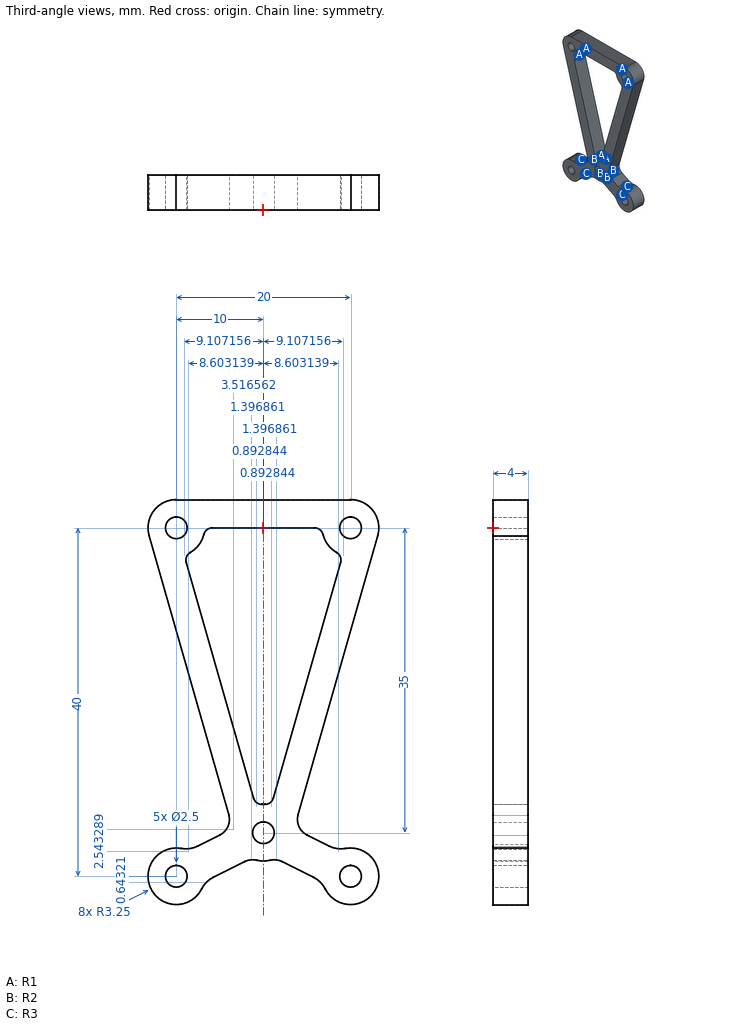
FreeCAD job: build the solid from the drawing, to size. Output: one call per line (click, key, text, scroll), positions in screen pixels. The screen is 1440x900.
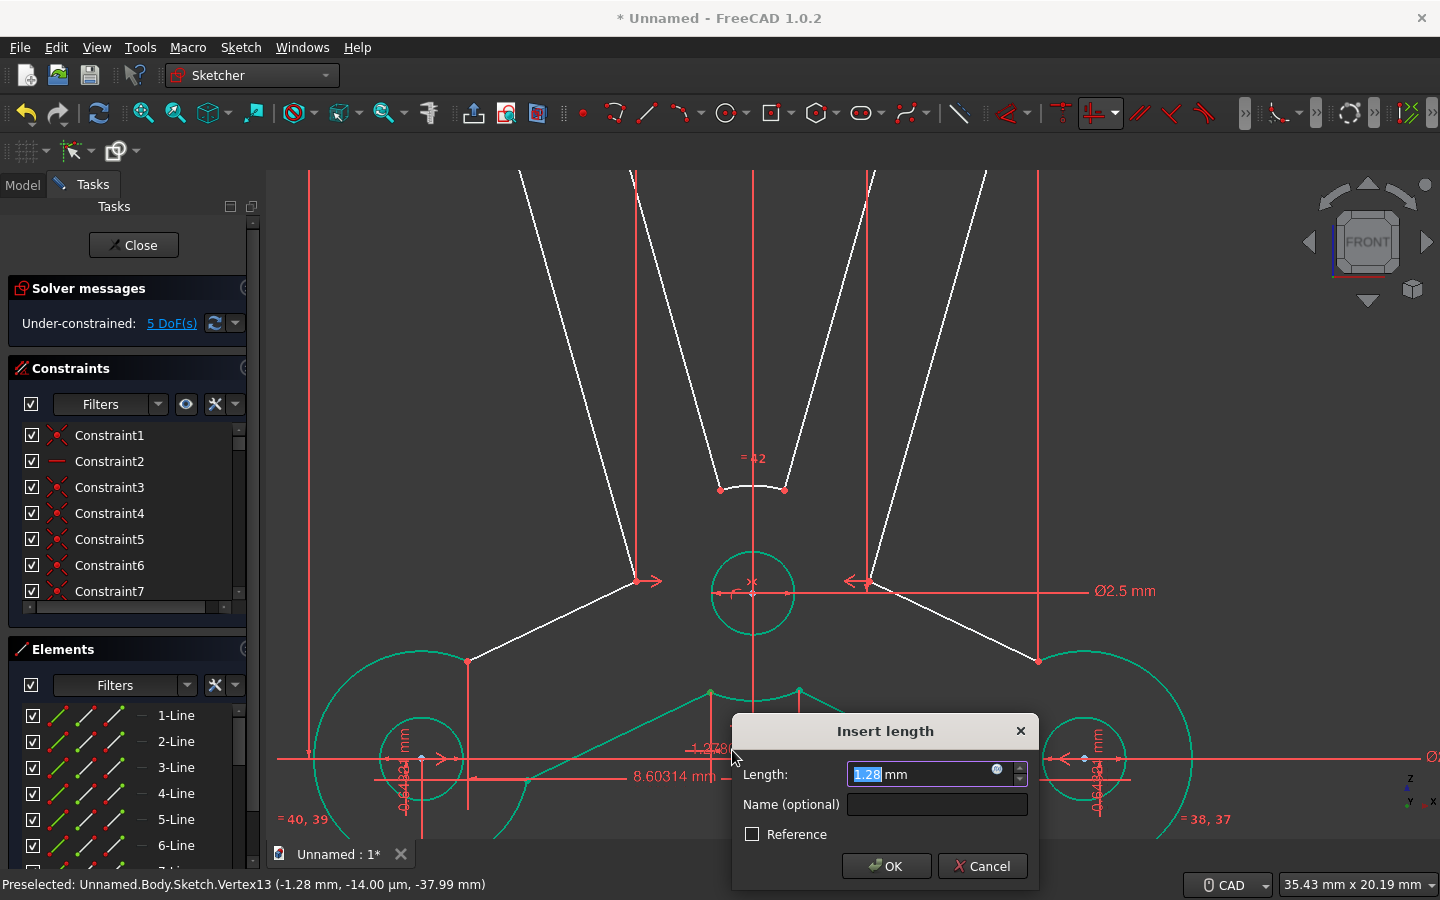
text(1.396861)
key(Return)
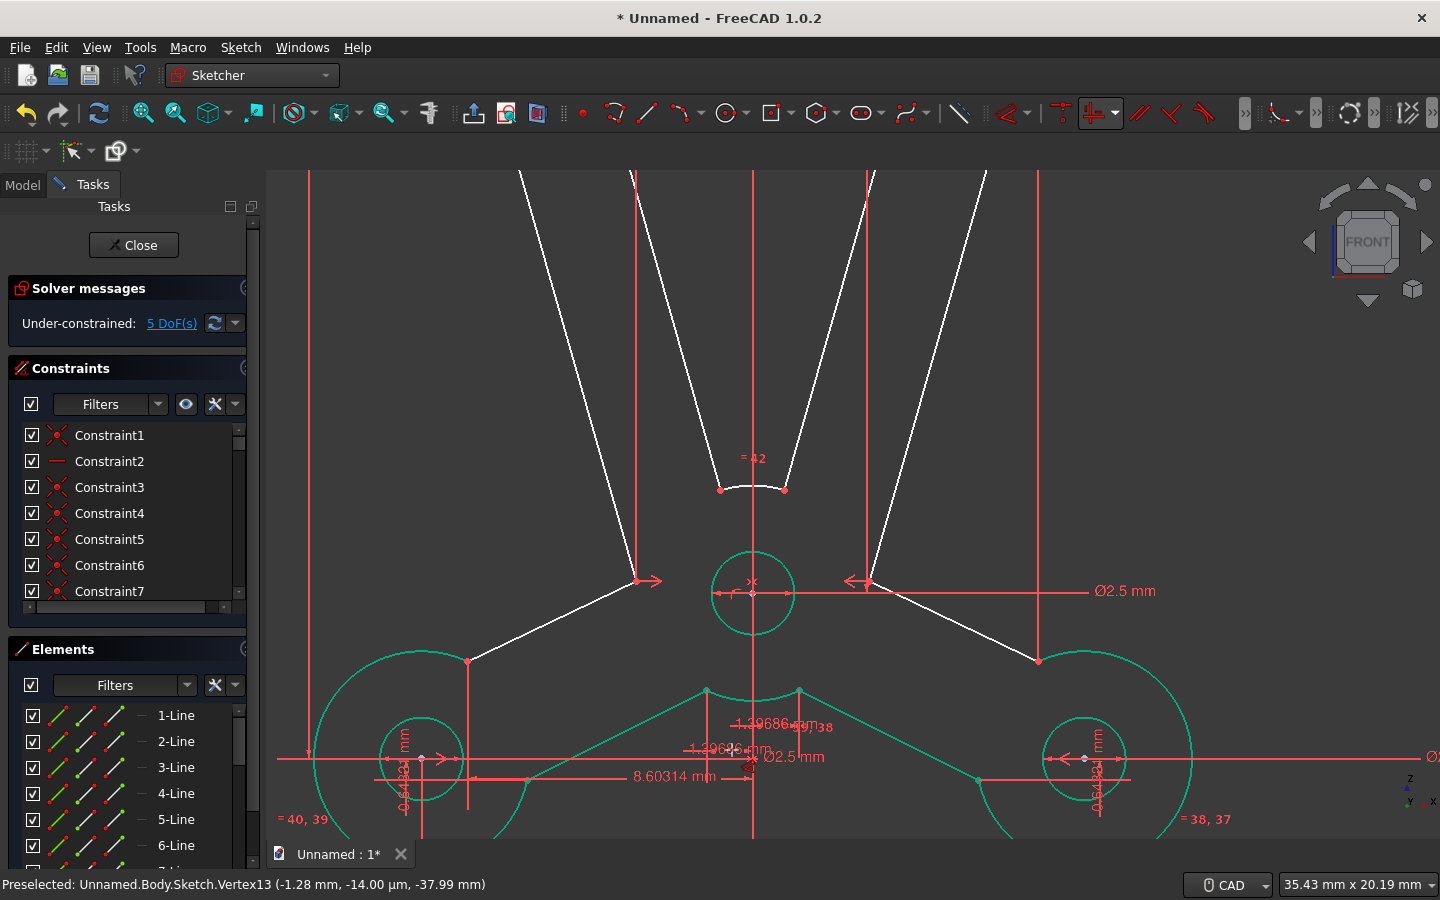
scroll(784, 490, up, 2)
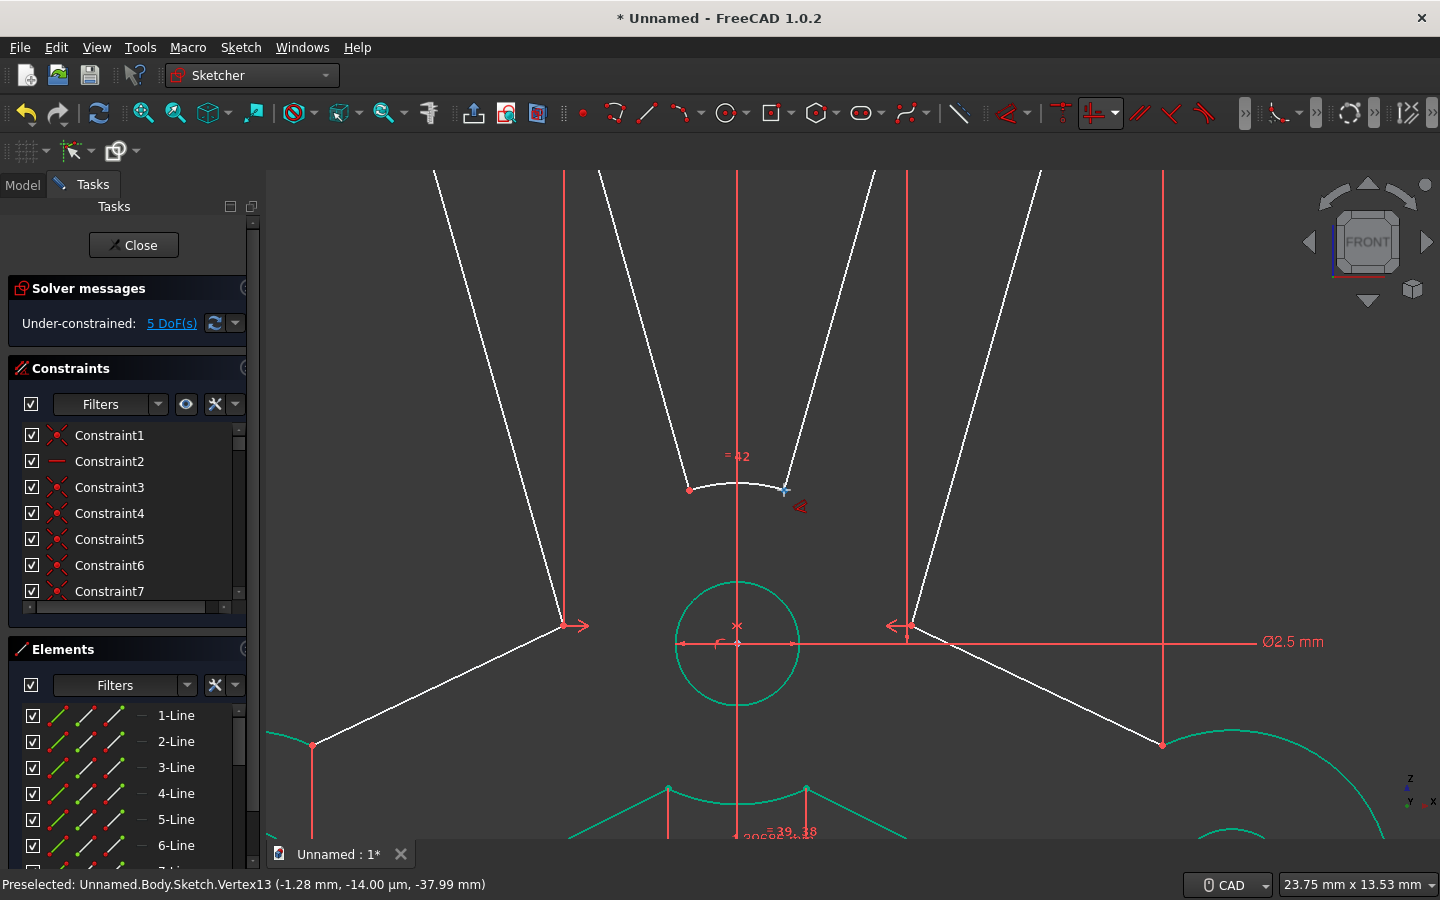
click(784, 490)
click(761, 524)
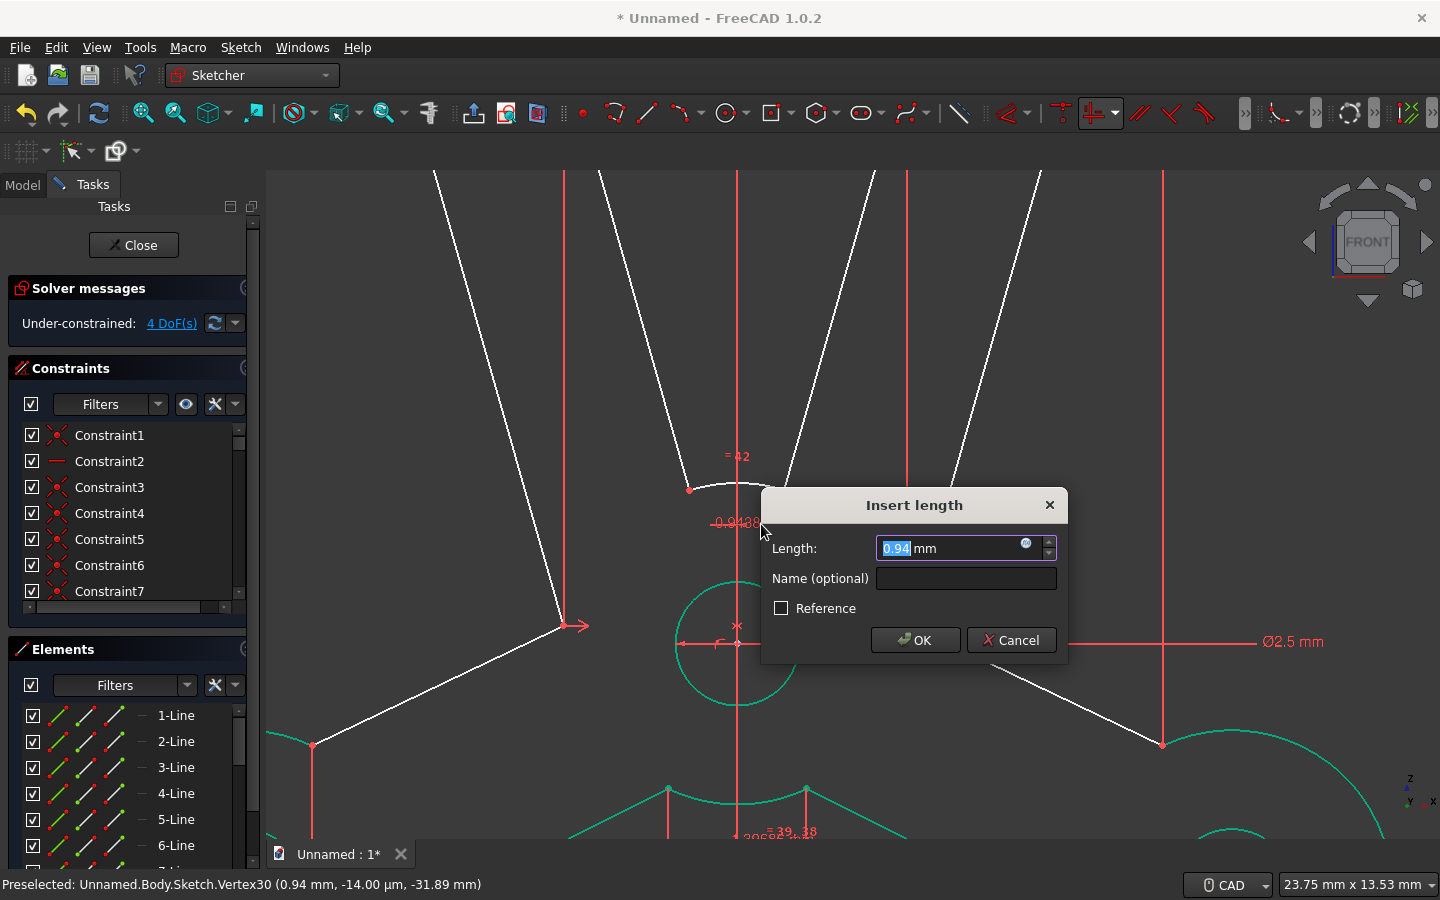
text(0.892844)
key(Return)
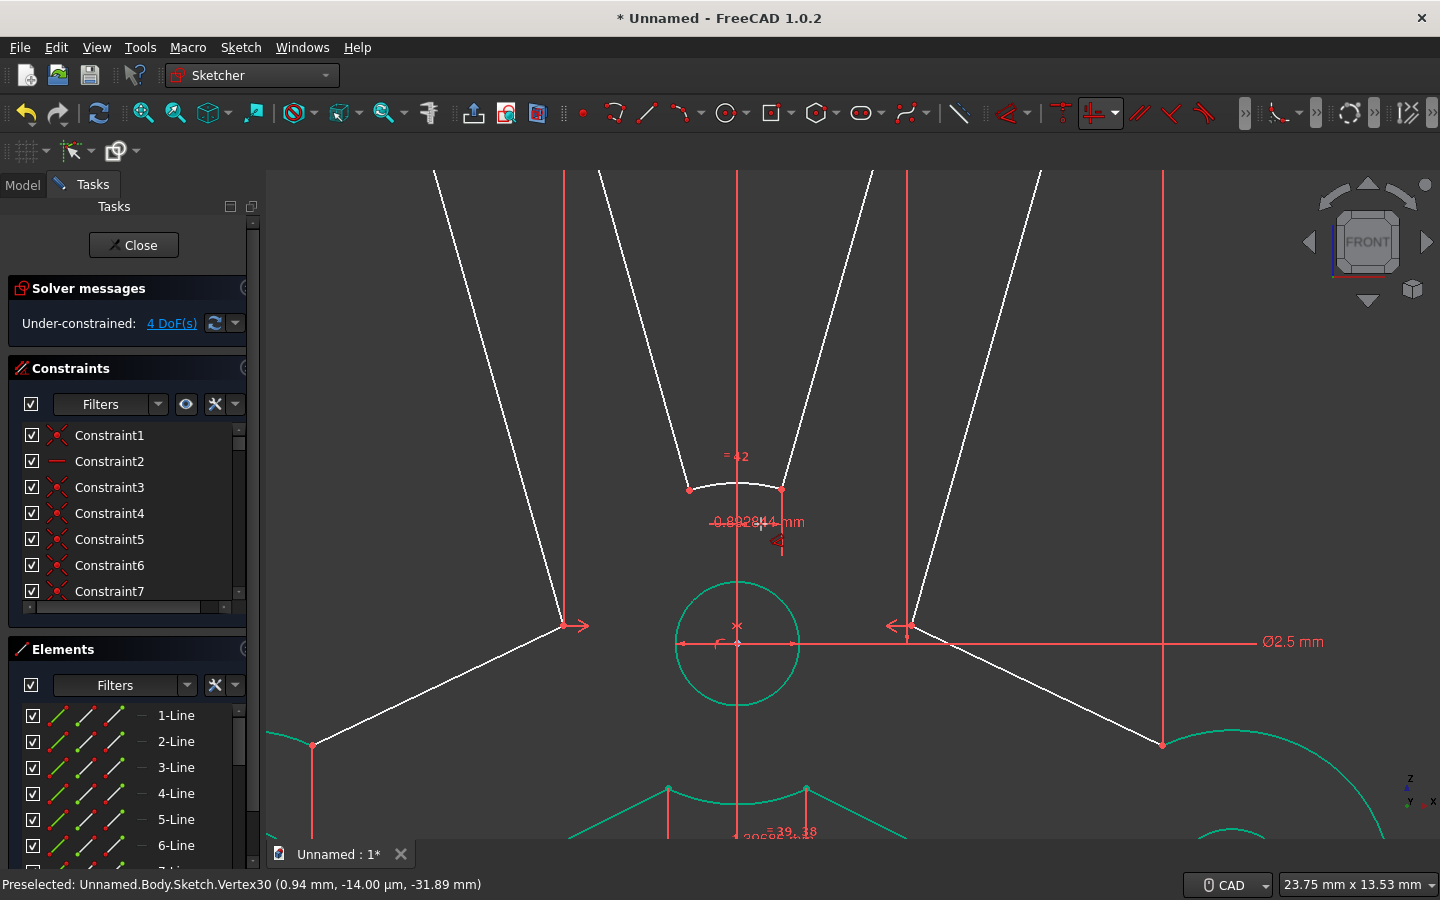
scroll(796, 668, down, 8)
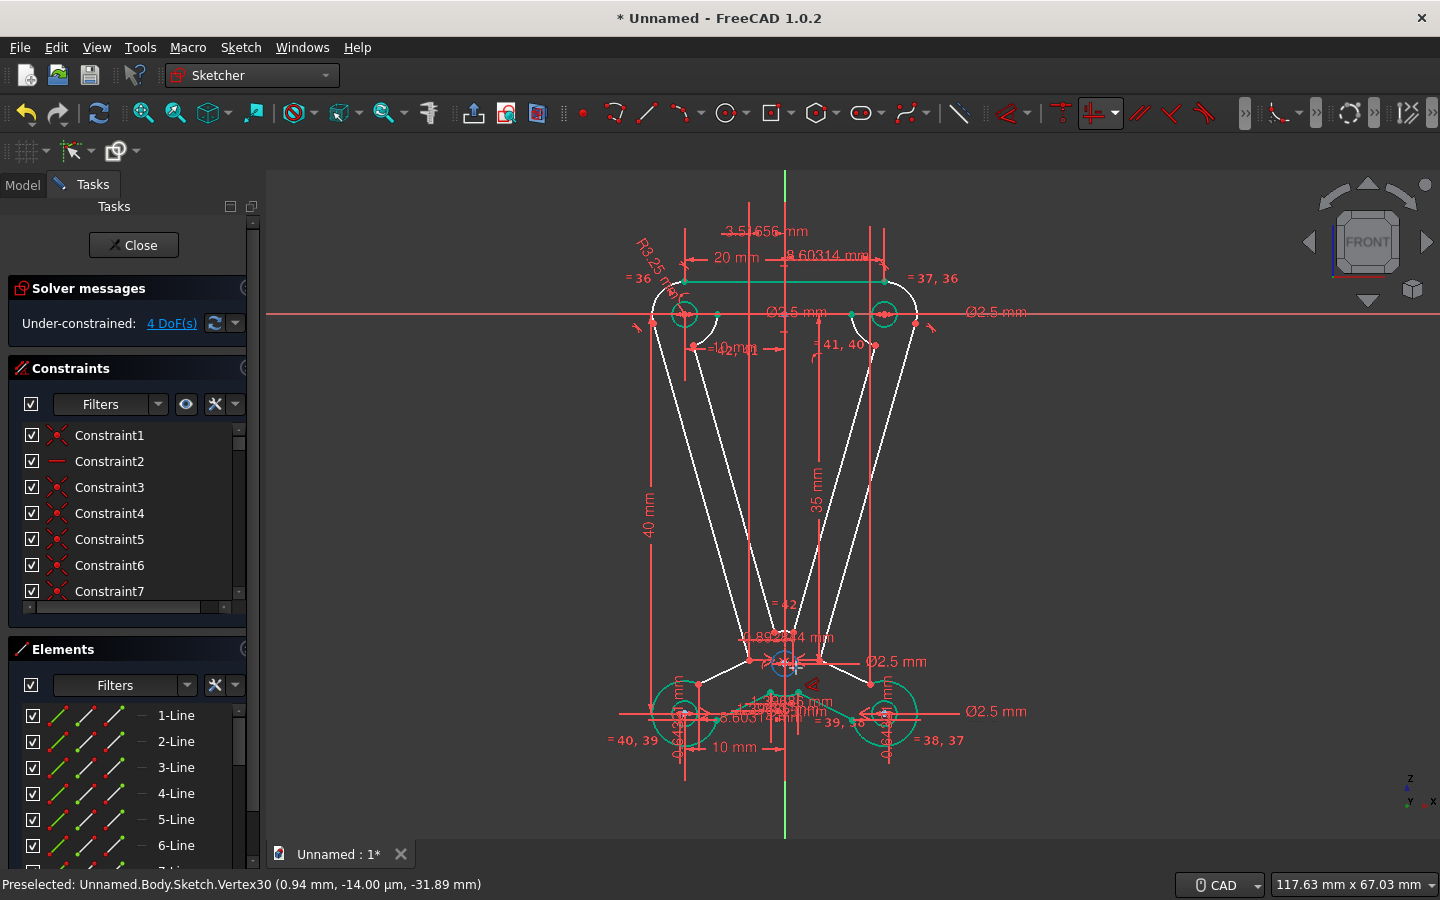
click(876, 346)
click(830, 380)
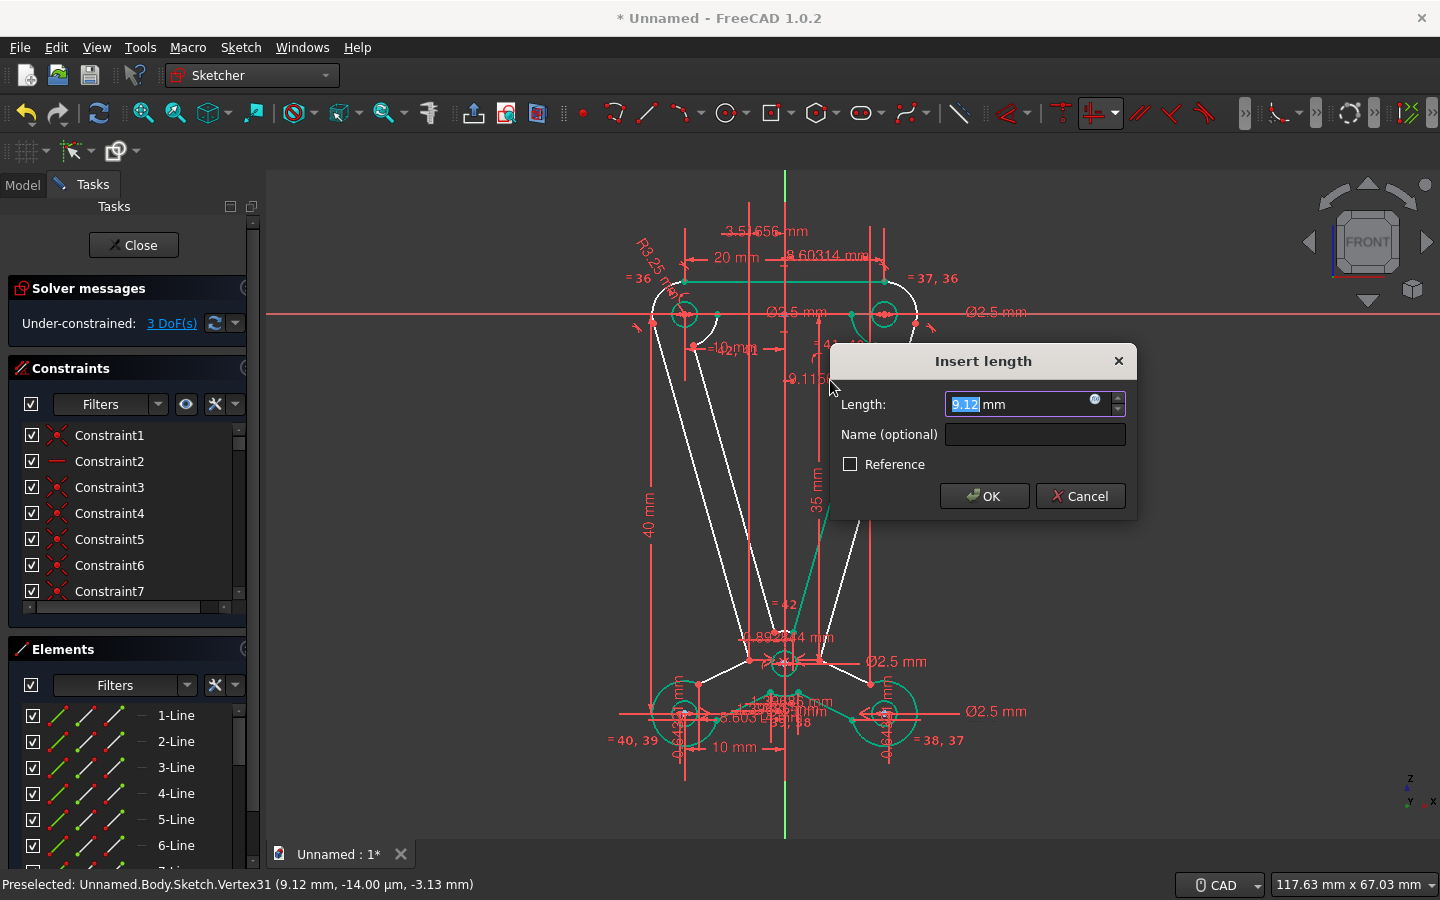
text(9.107156)
key(Return)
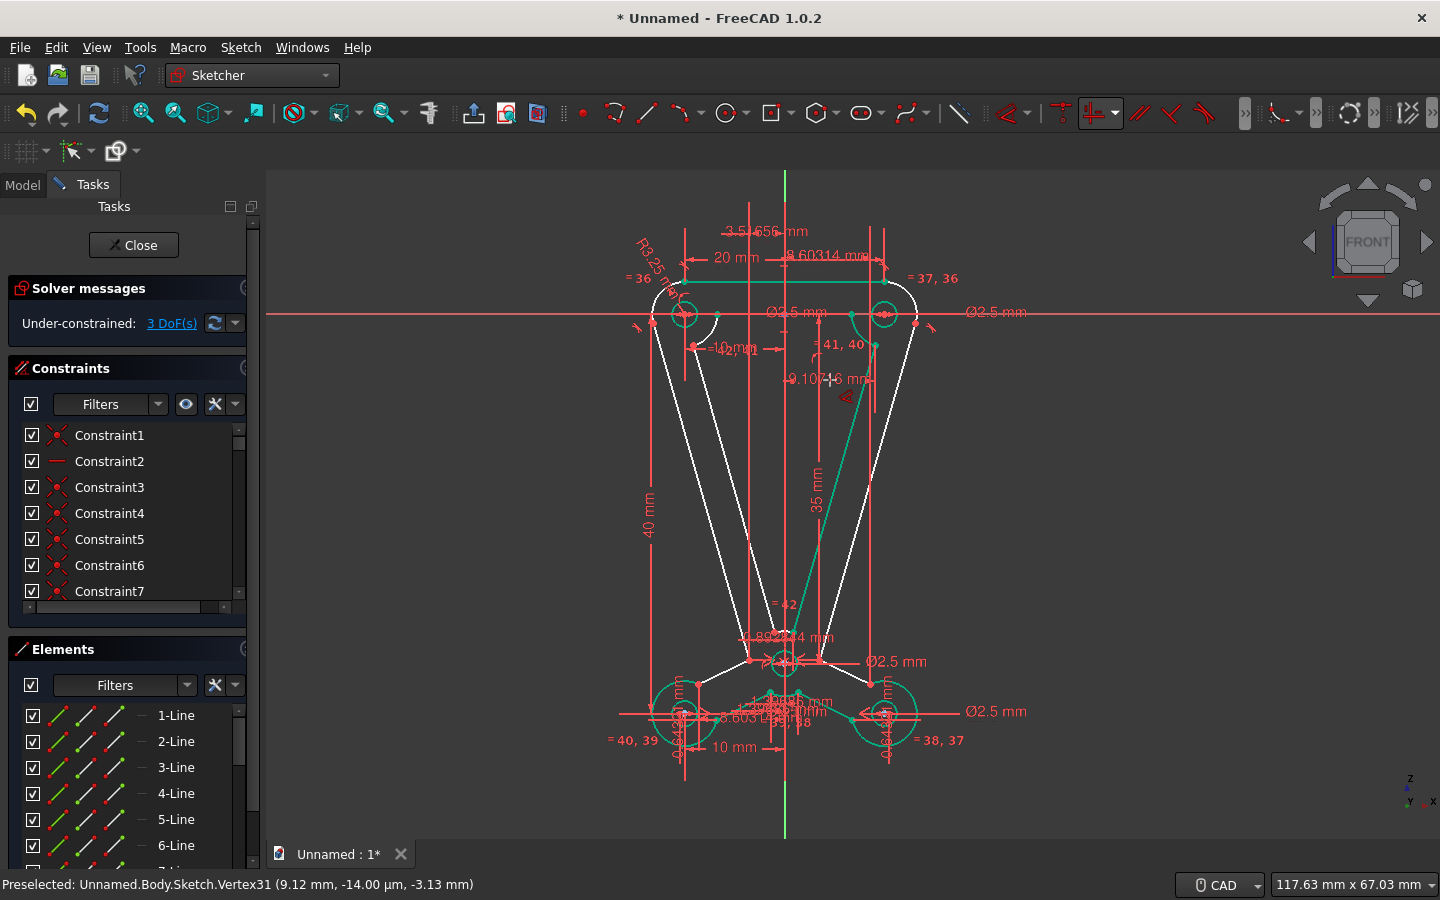
click(694, 346)
click(739, 380)